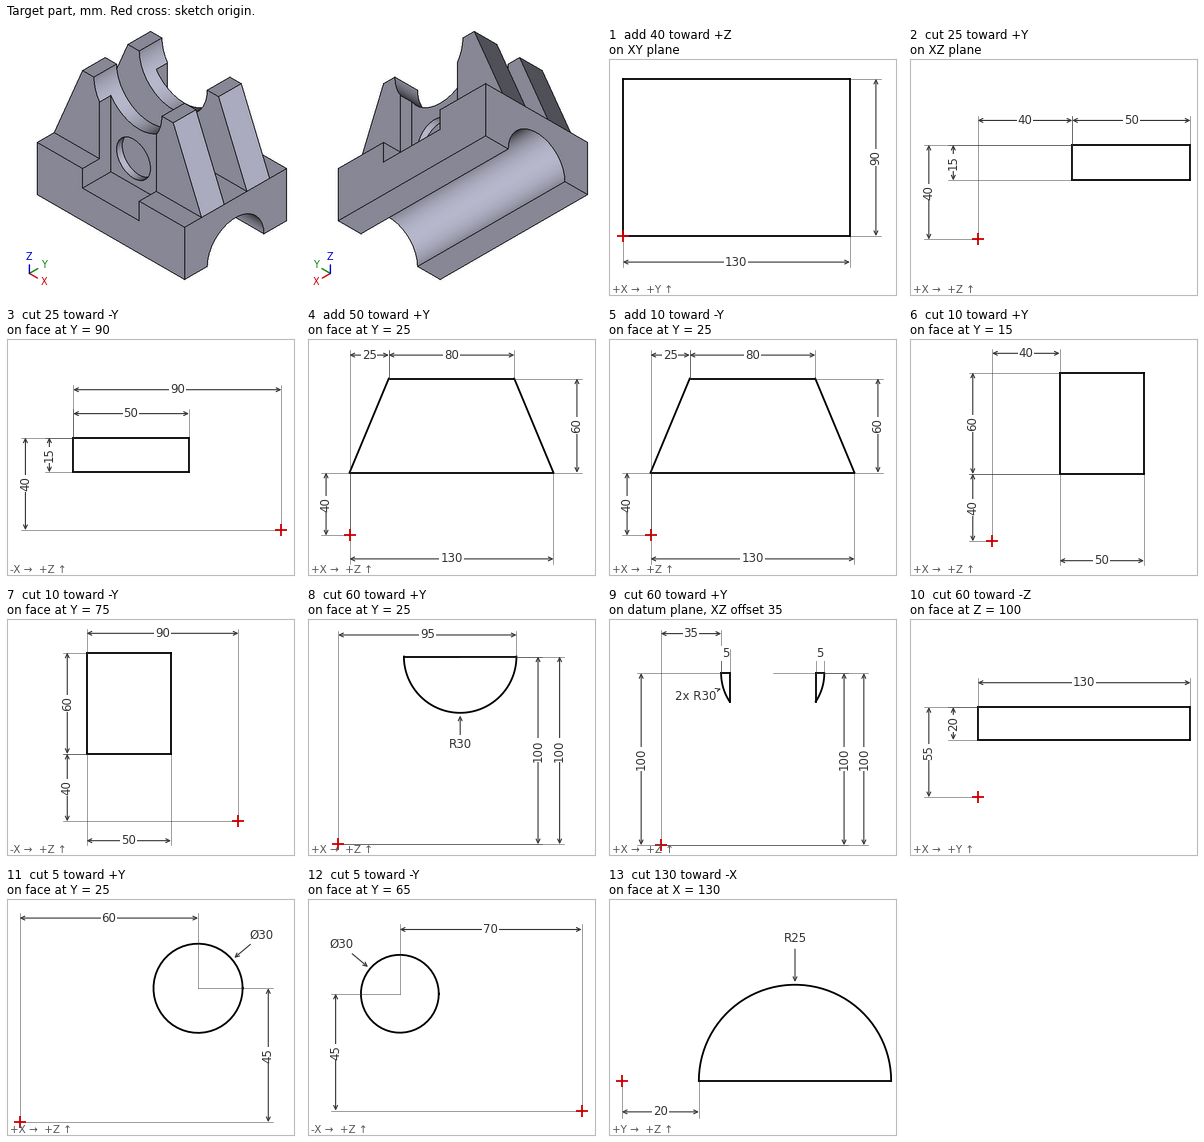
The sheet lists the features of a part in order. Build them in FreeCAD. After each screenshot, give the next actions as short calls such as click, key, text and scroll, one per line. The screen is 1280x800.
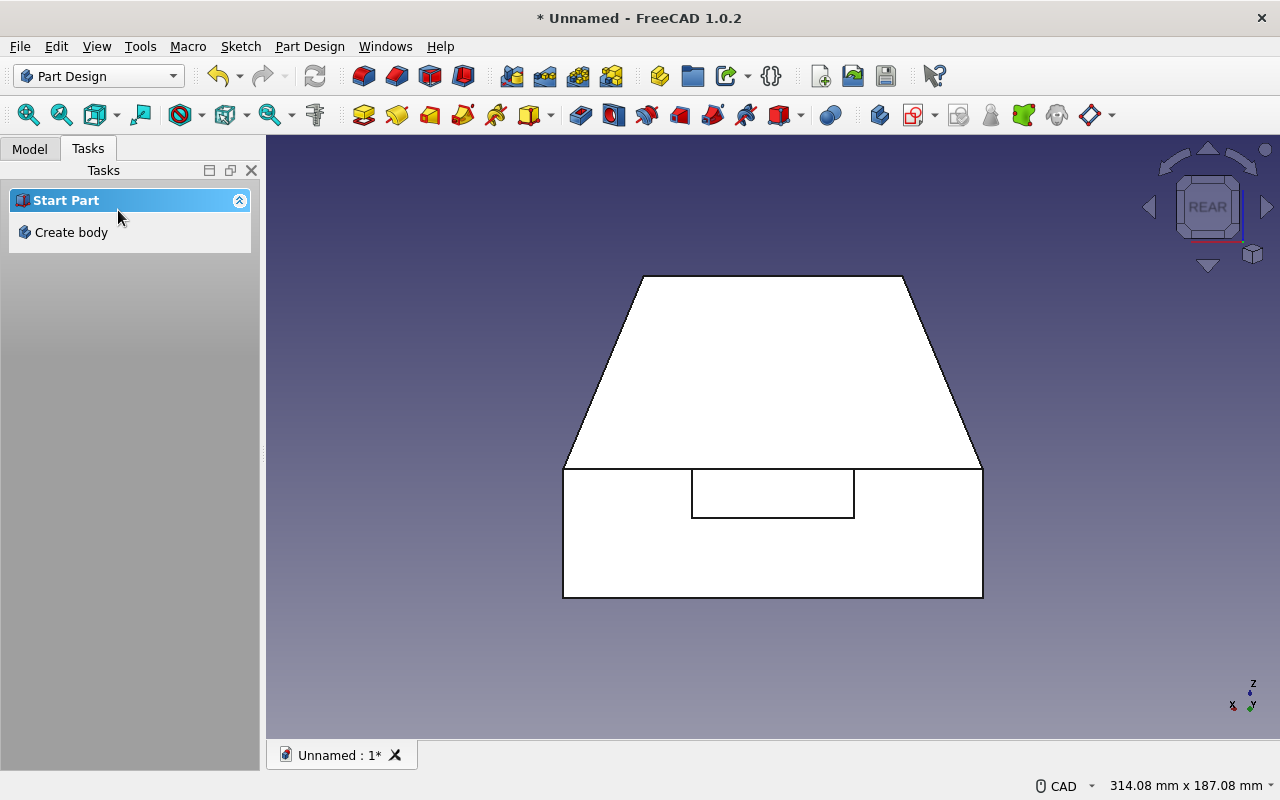
click(713, 371)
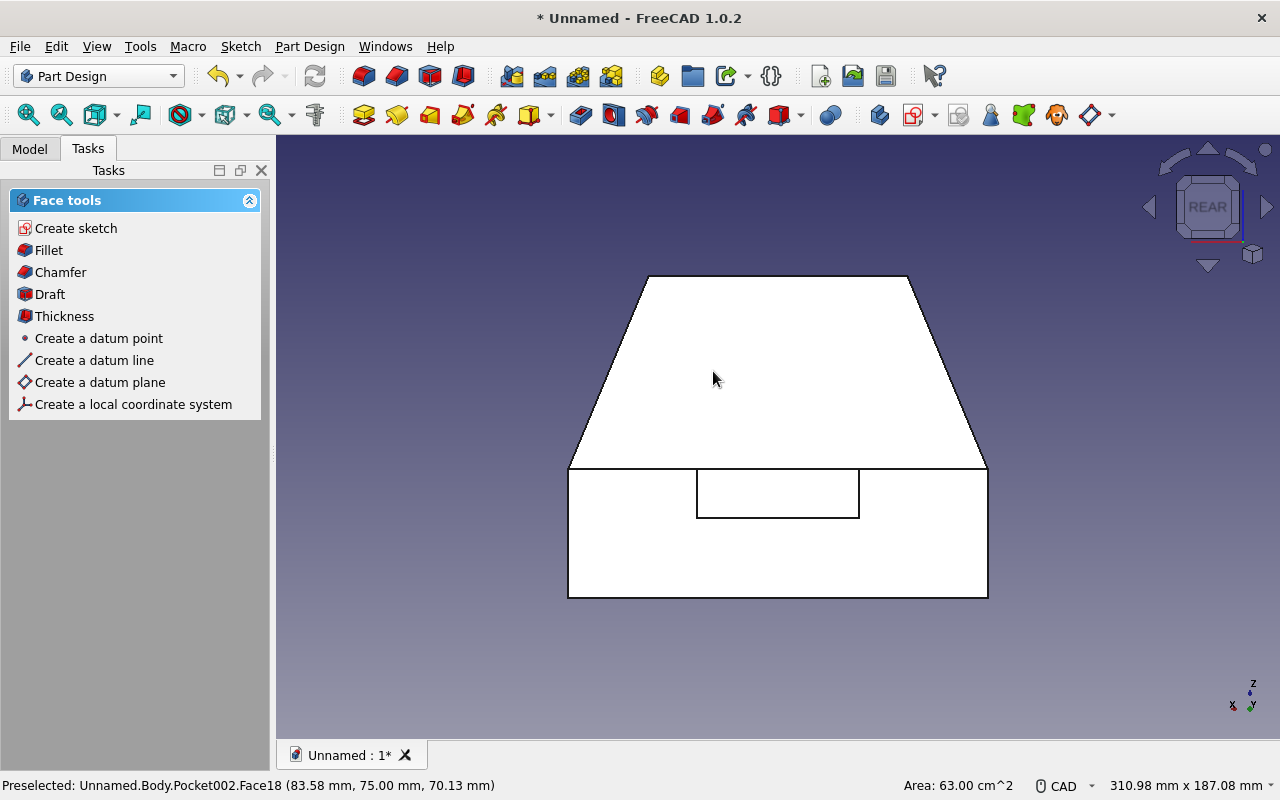
click(912, 116)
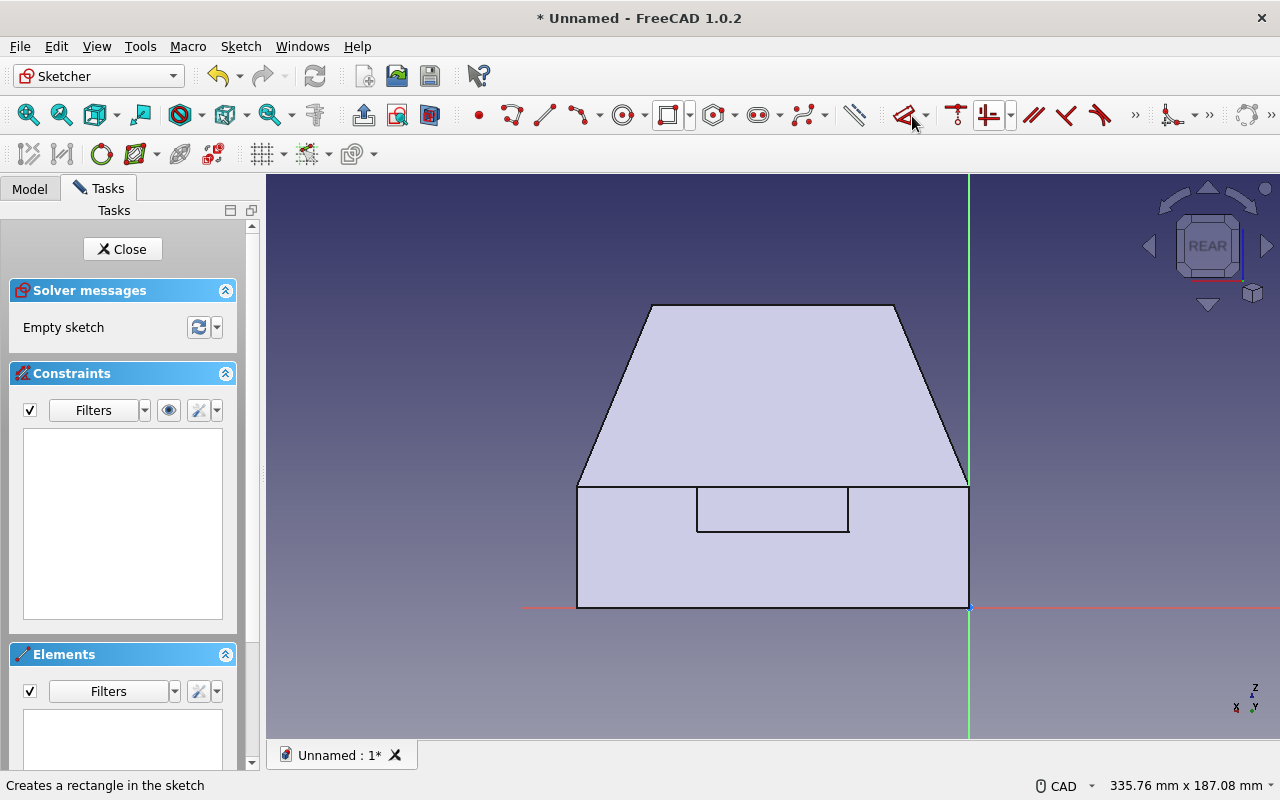
click(430, 116)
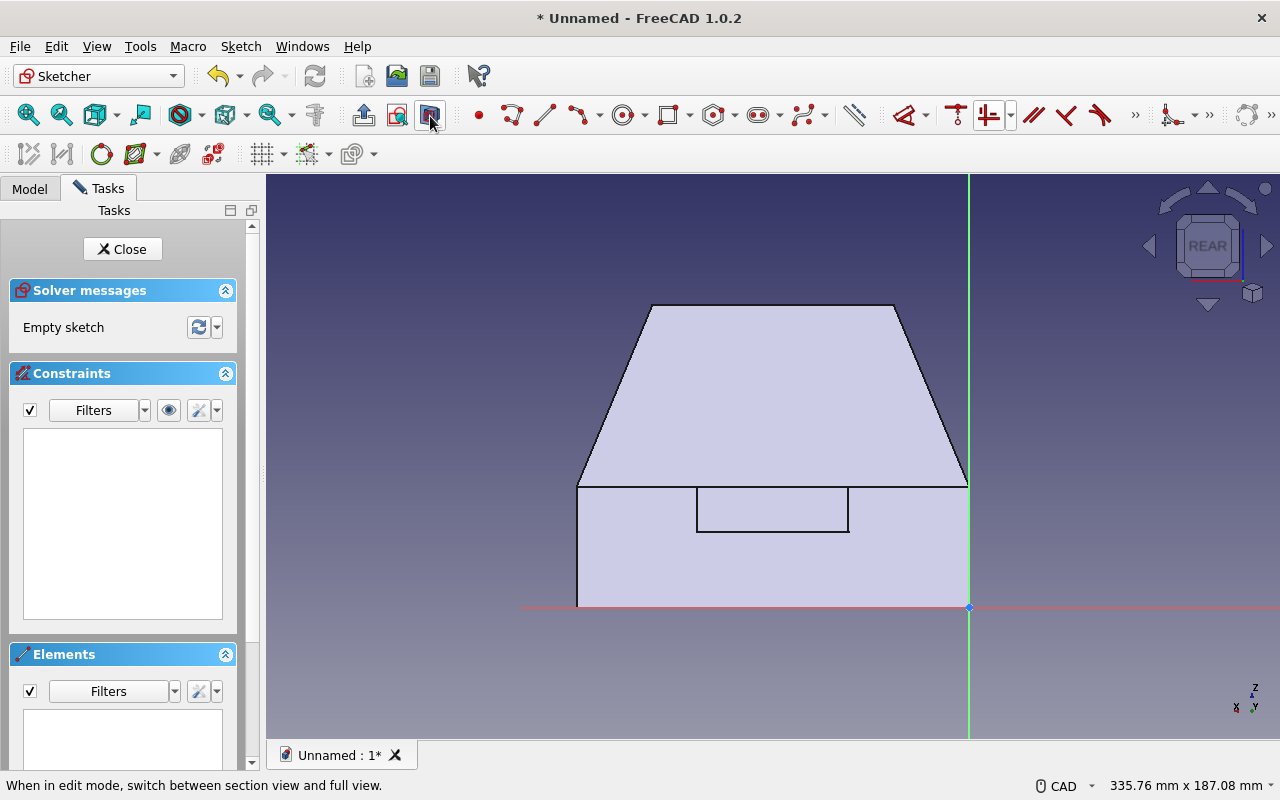
key(g)
key(r)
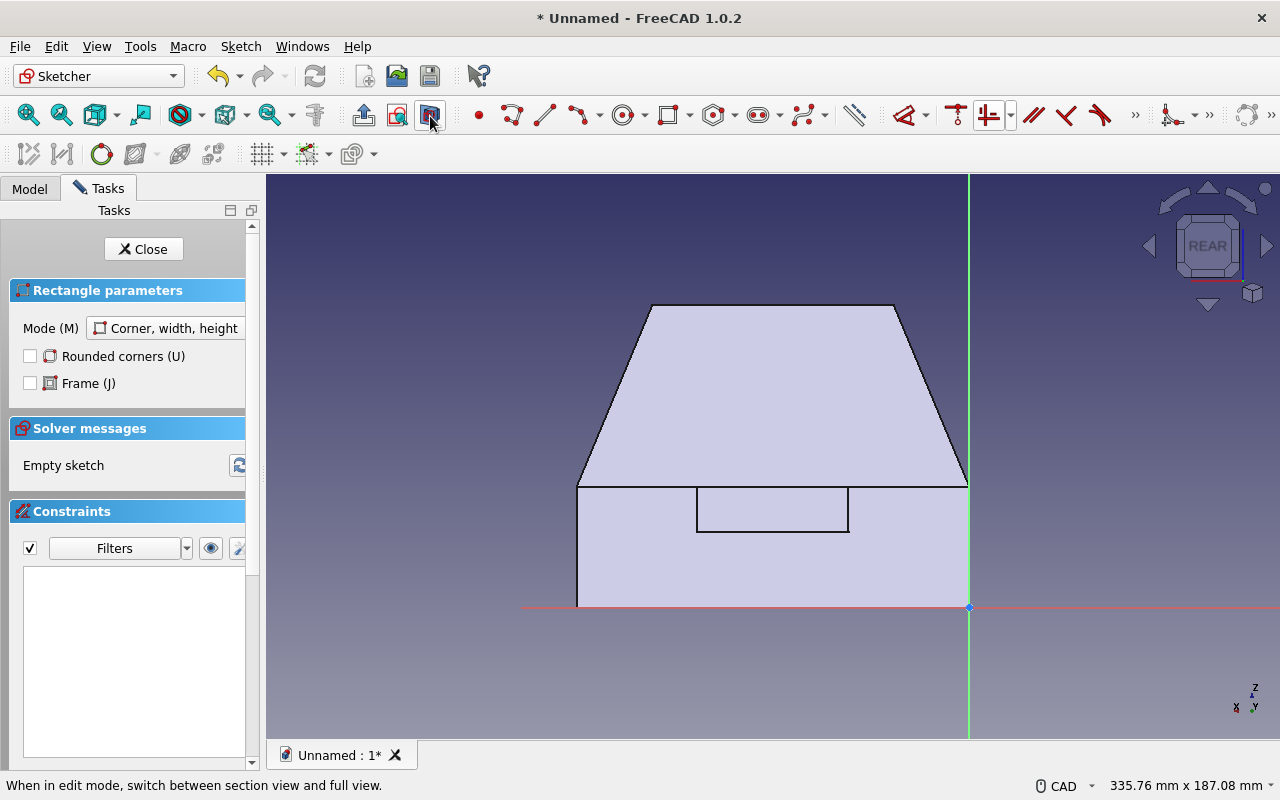
click(697, 305)
click(849, 487)
key(Escape)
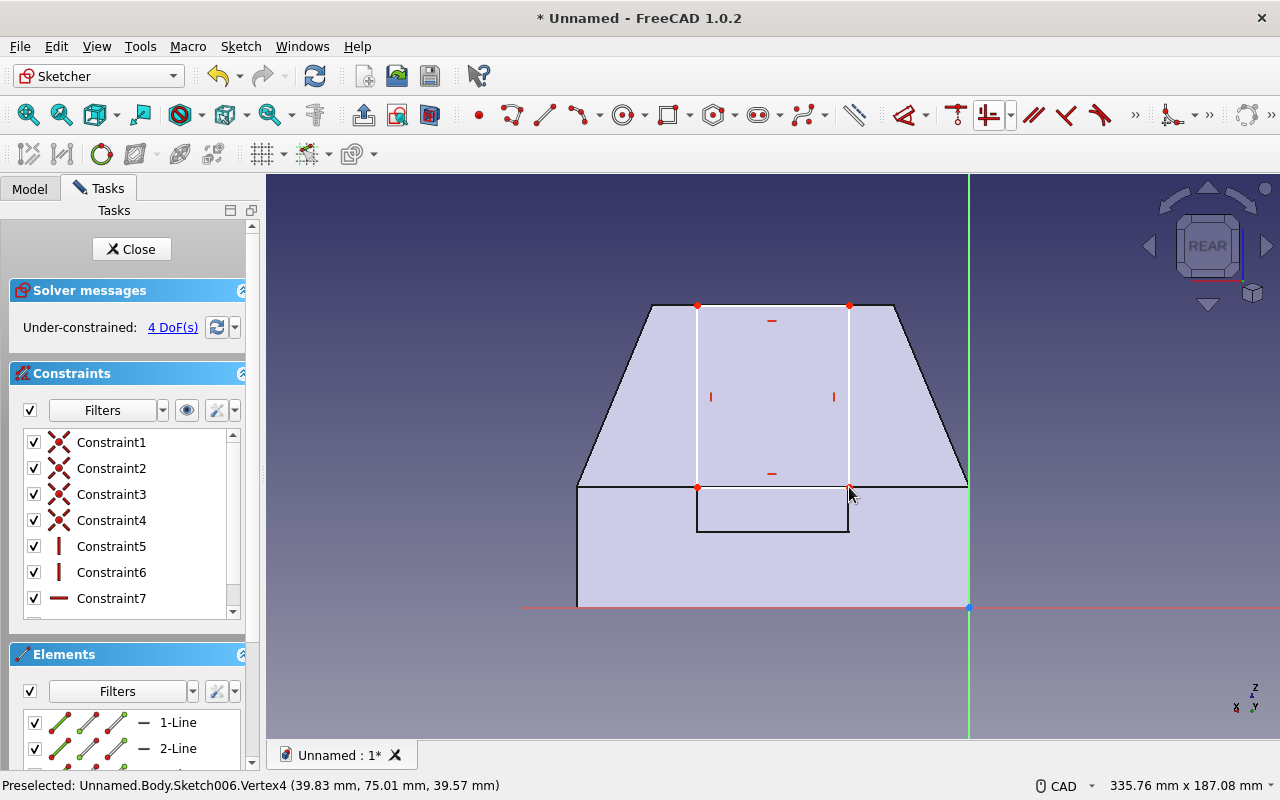
click(904, 116)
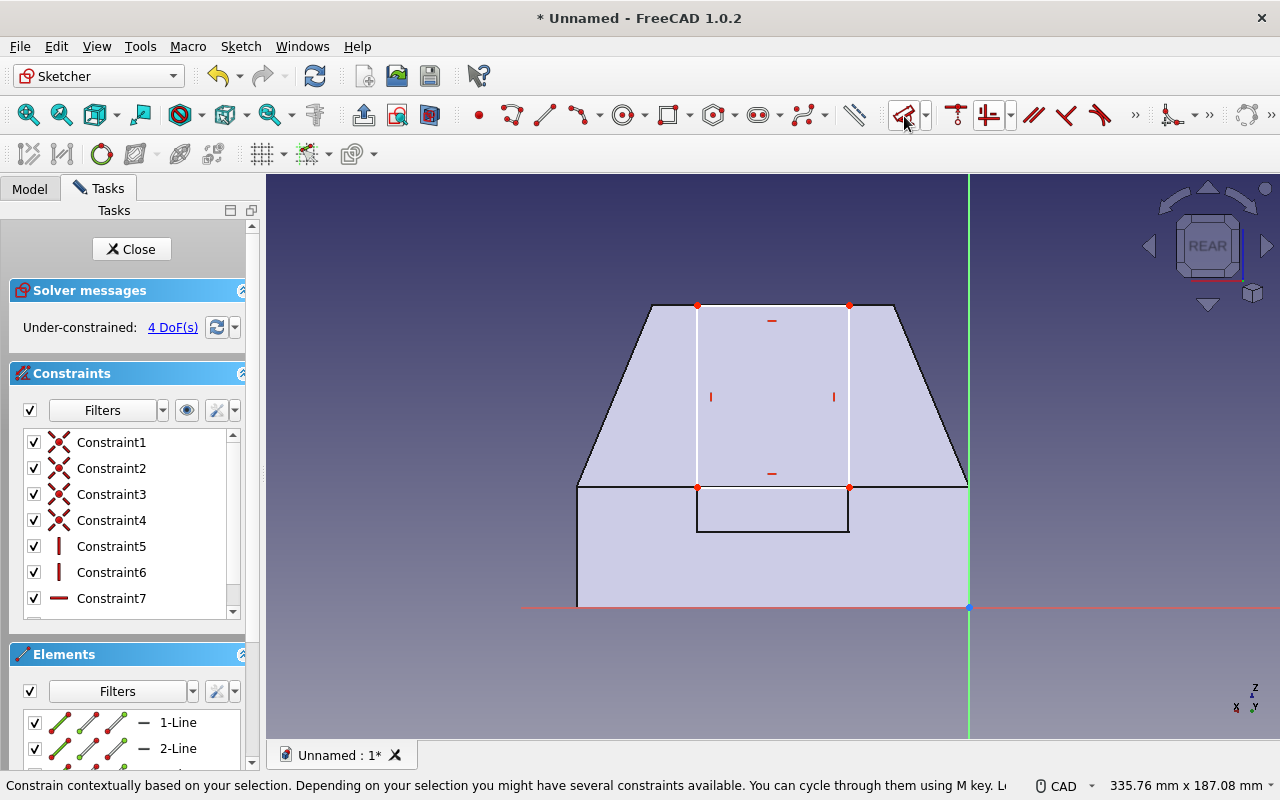
click(697, 361)
click(663, 397)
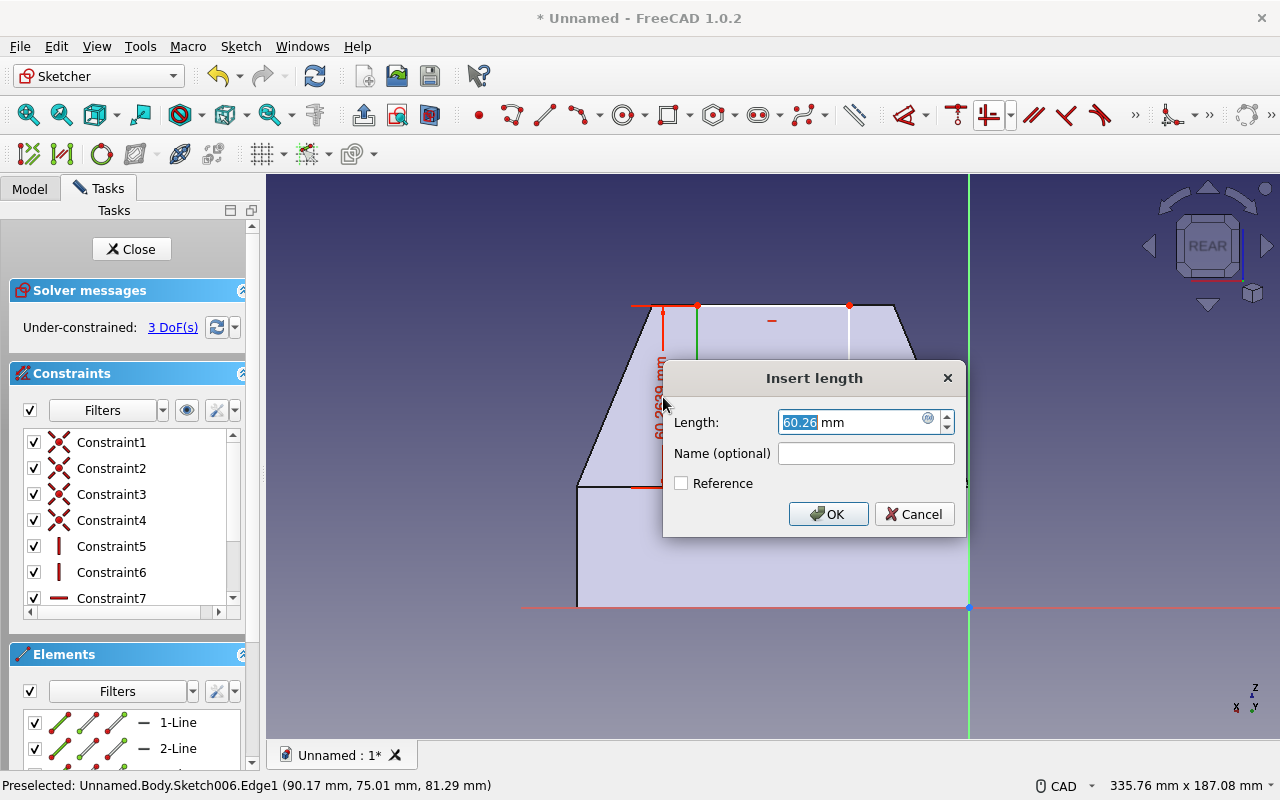
text(60)
key(Return)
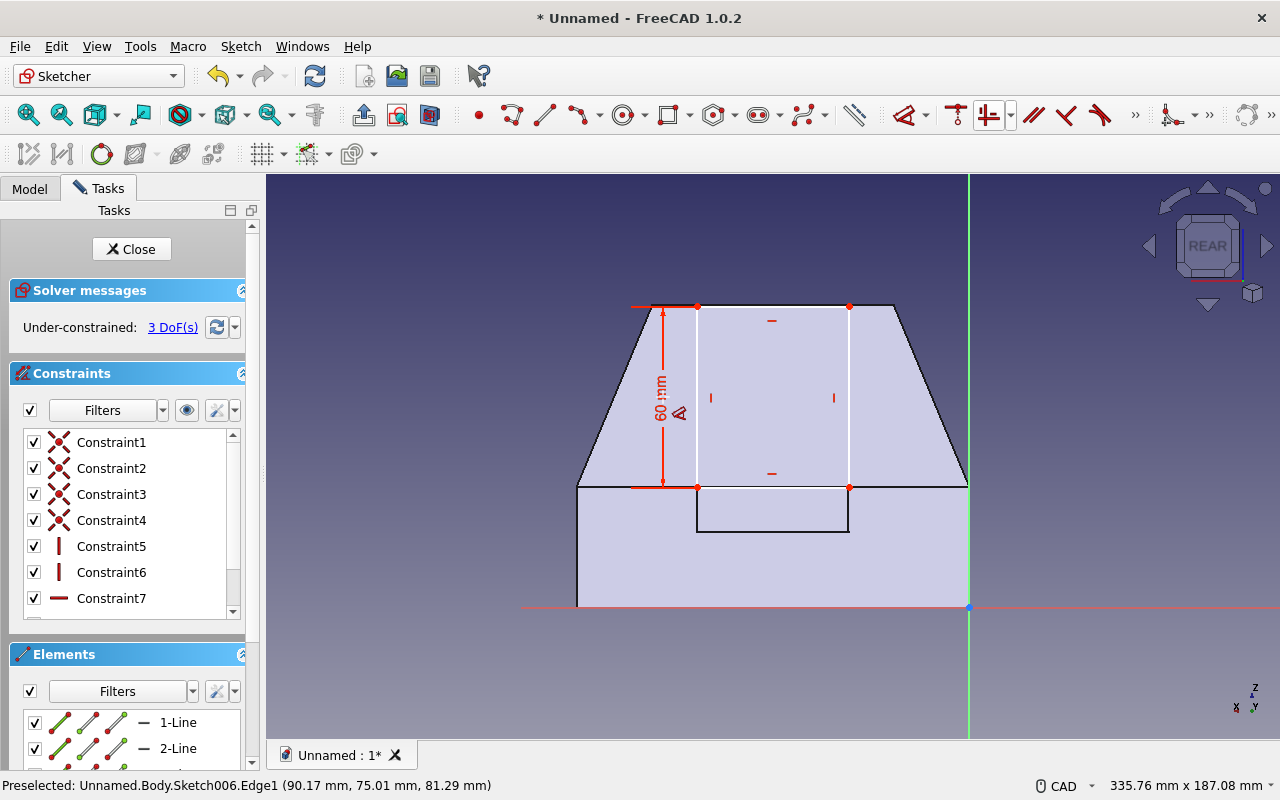
click(743, 488)
click(773, 522)